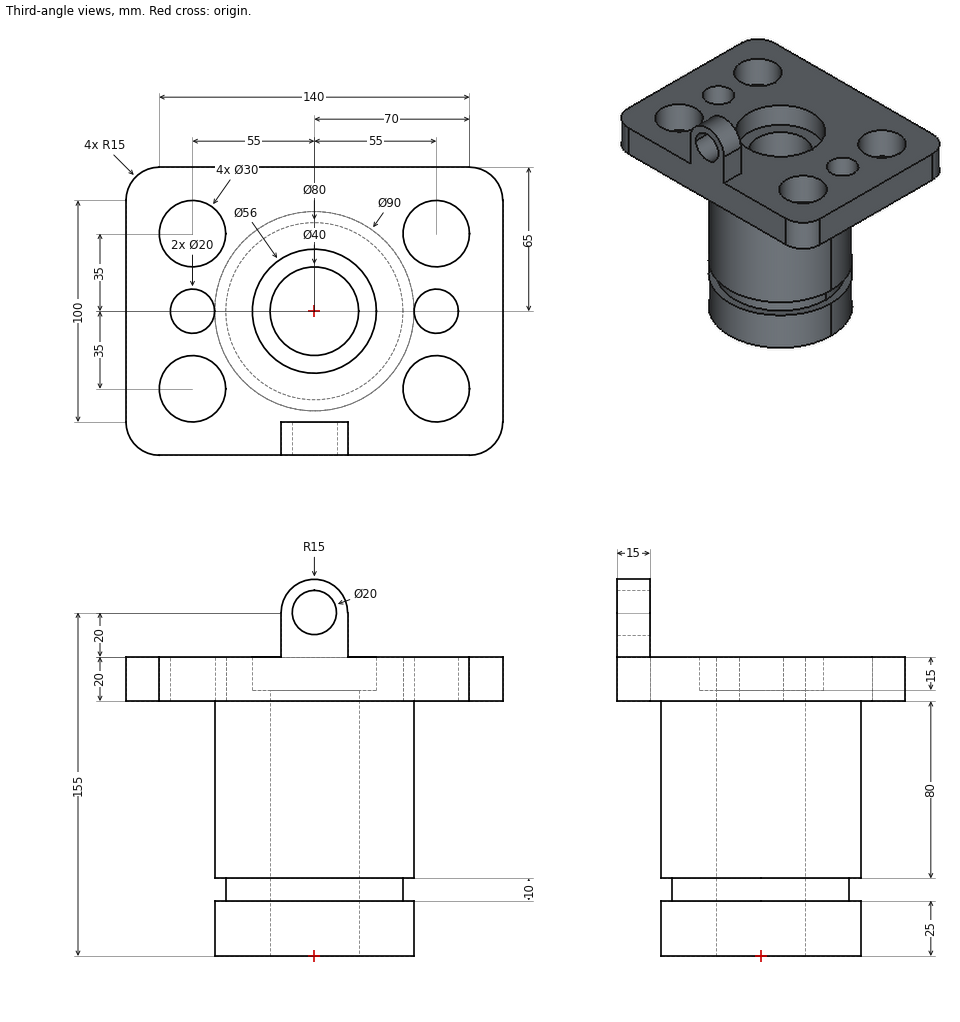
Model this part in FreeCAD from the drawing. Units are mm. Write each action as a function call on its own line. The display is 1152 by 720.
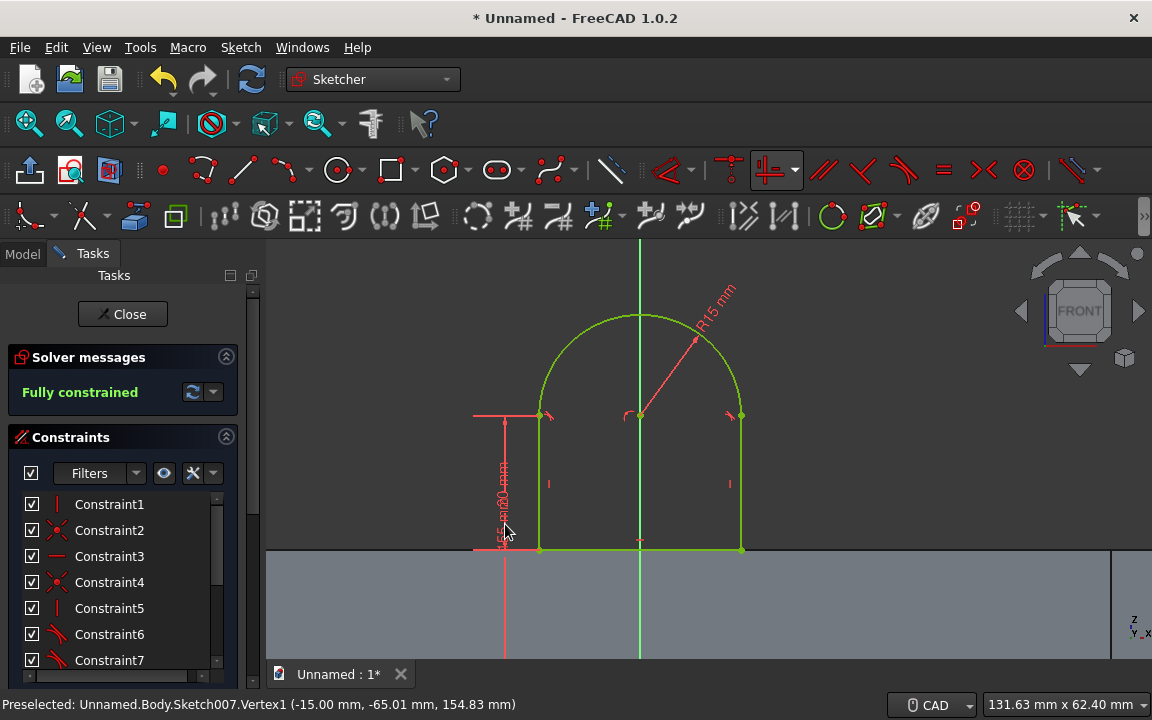
click(123, 314)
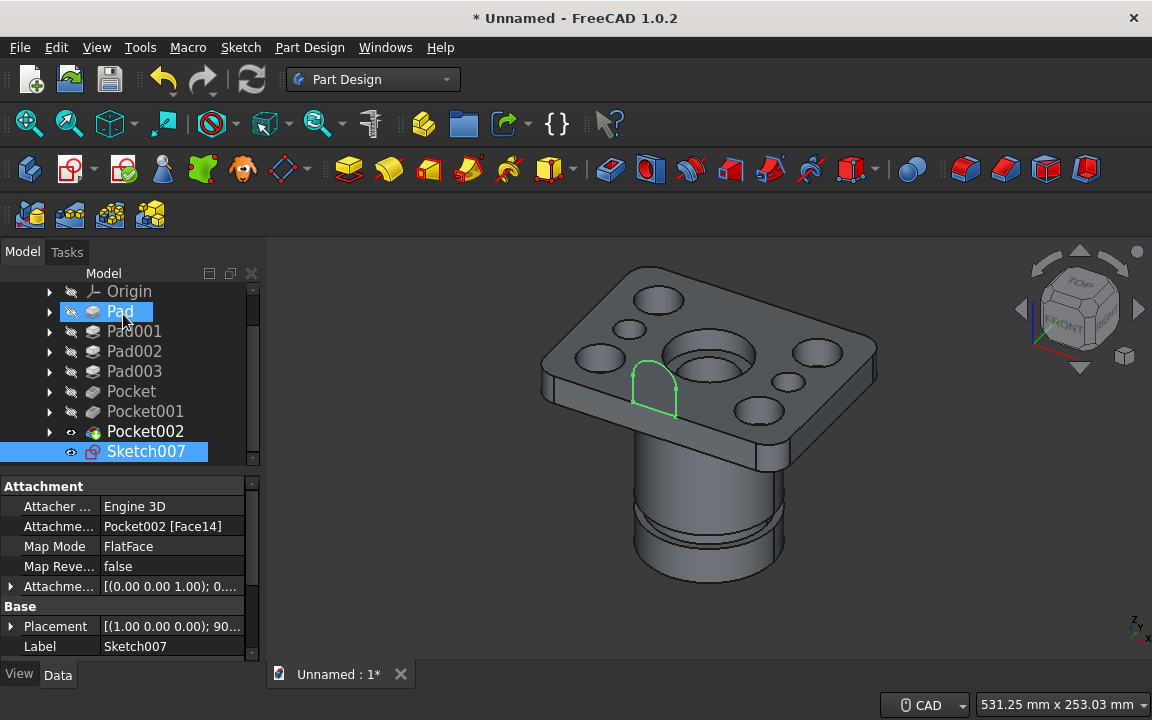
click(350, 170)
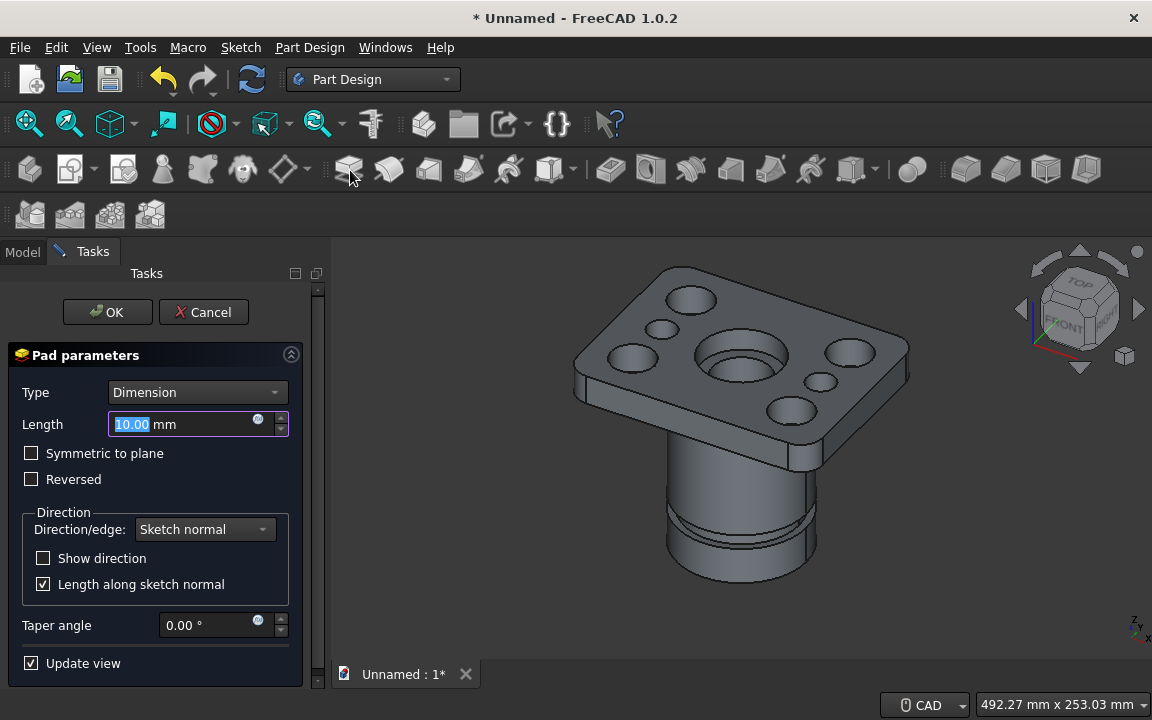
text(15)
key(Tab)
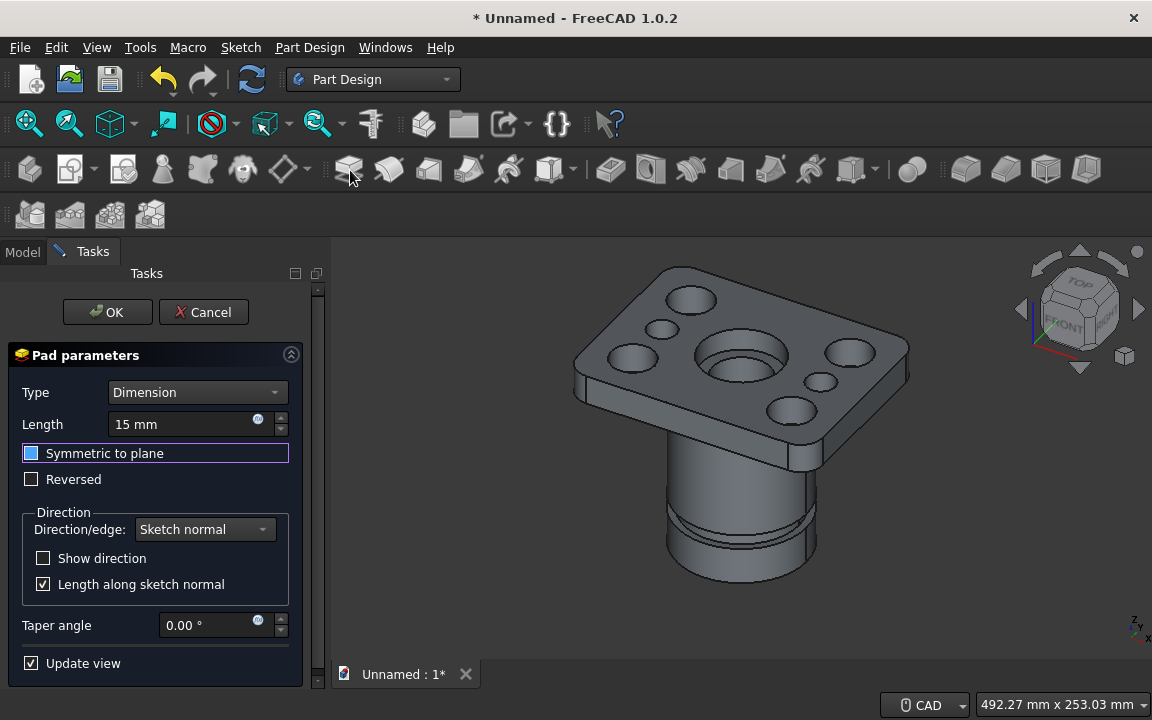
click(30, 479)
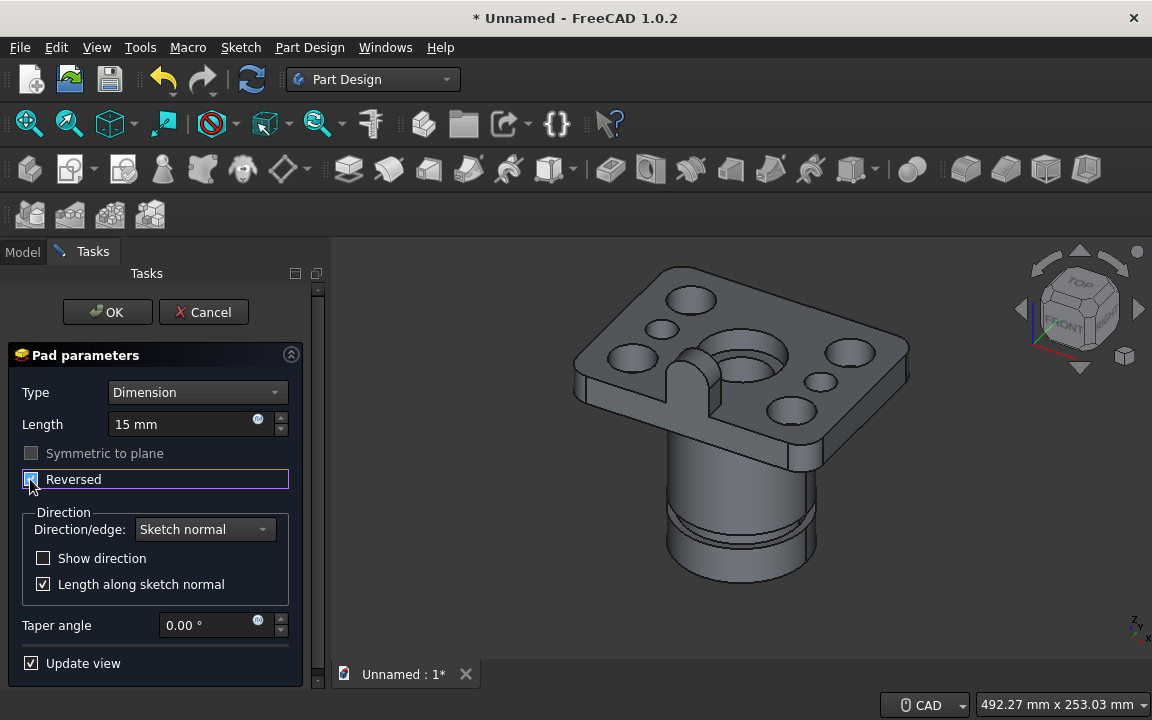
click(108, 312)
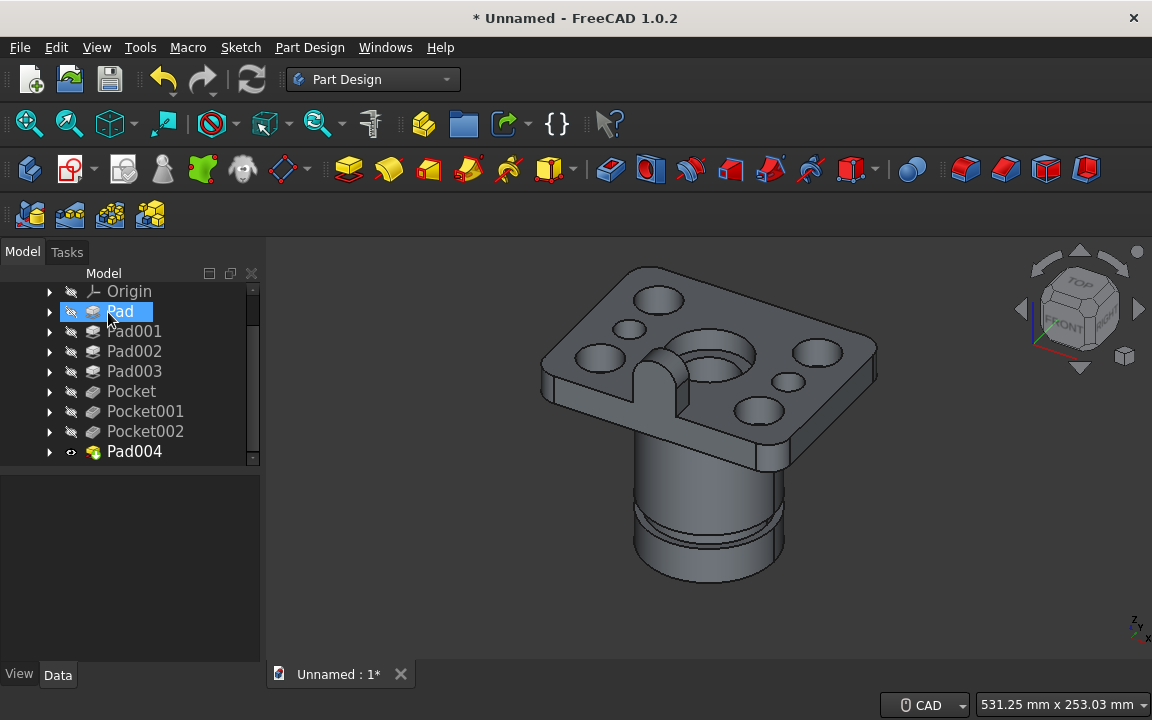
click(30, 124)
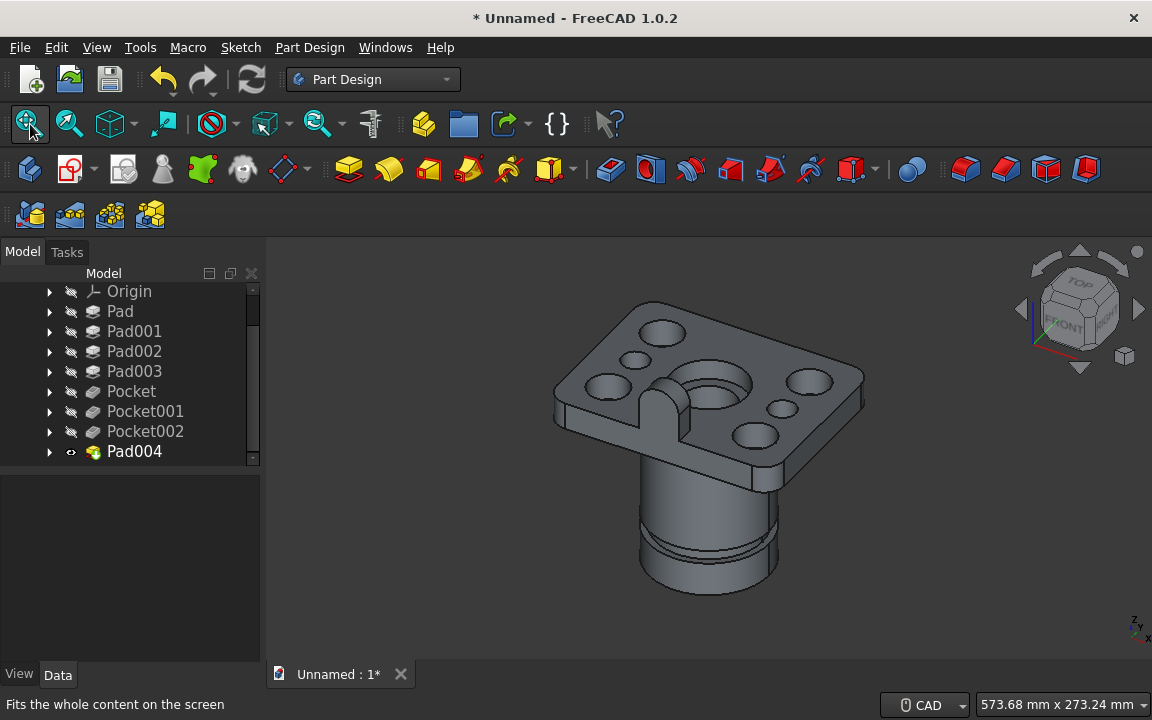
key(4)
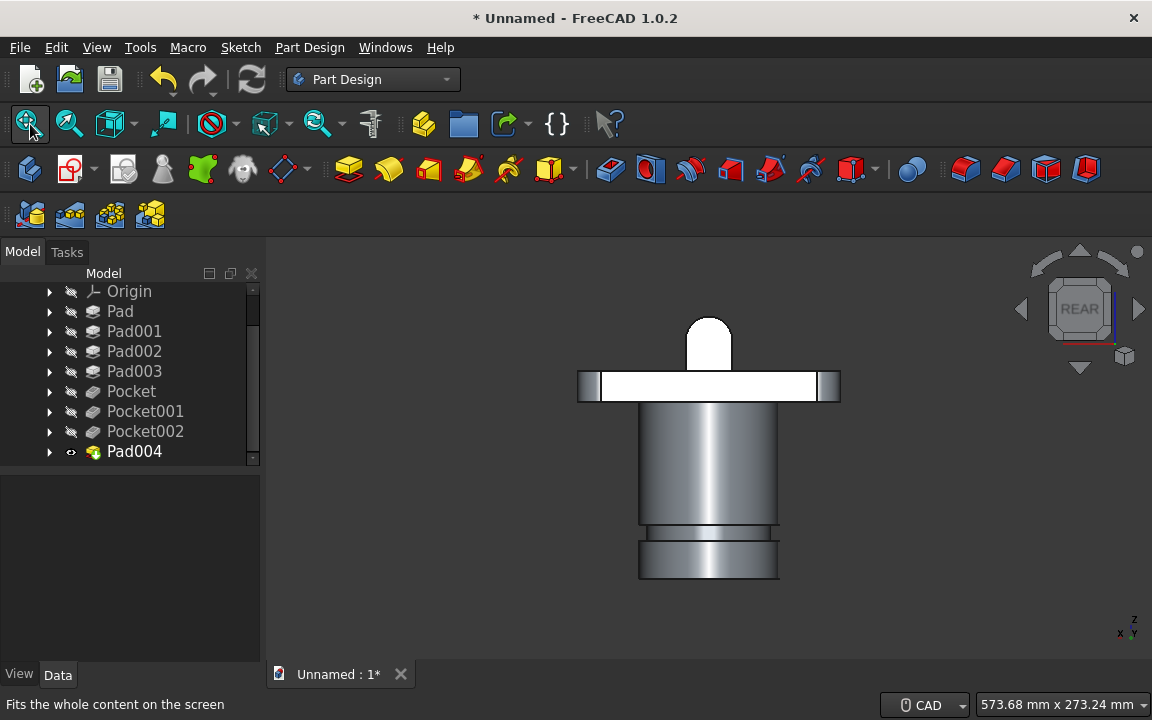
click(709, 343)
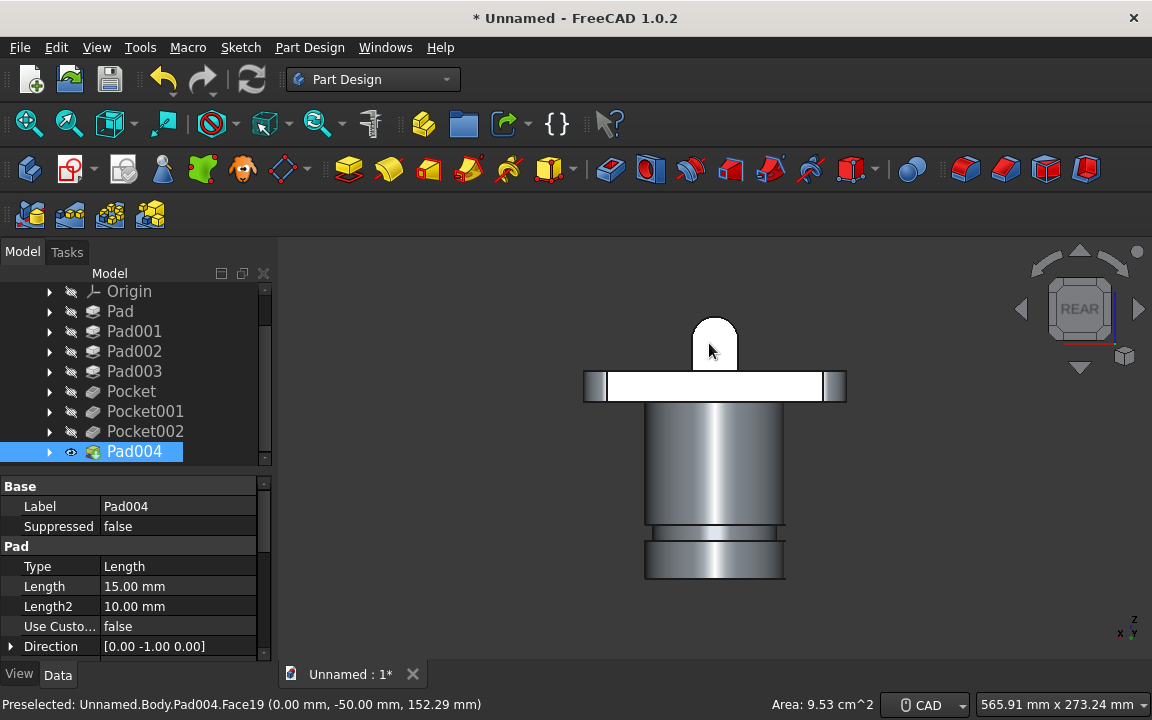
click(70, 170)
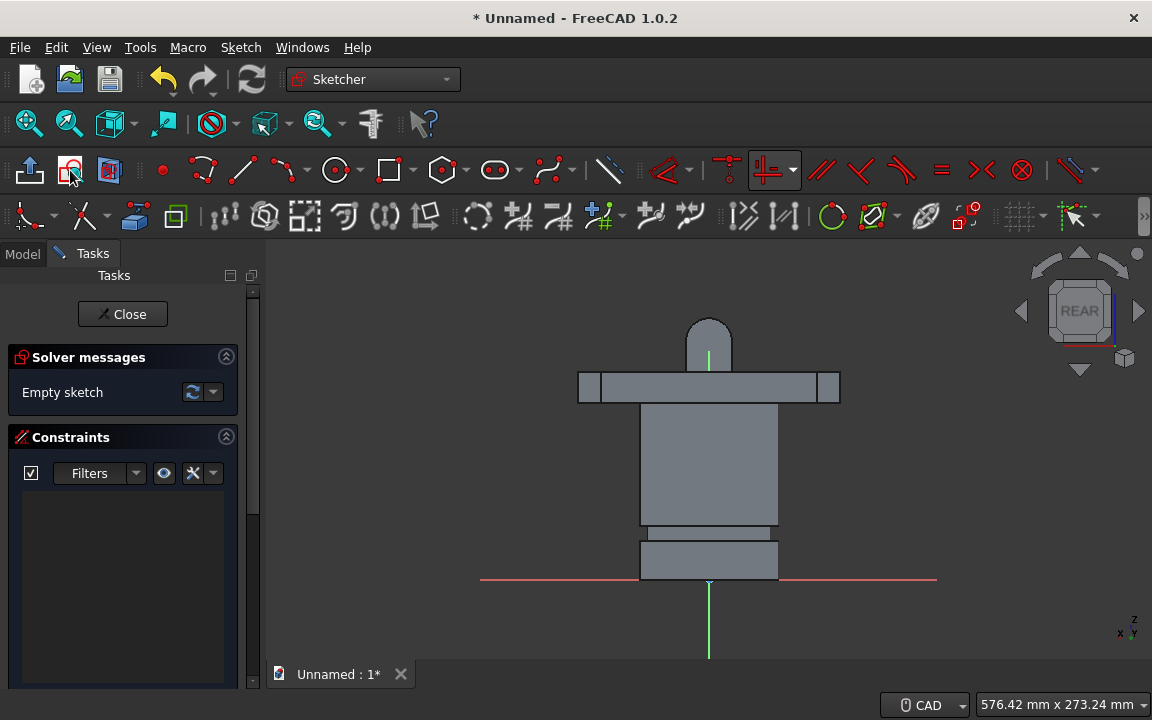
scroll(718, 328, up, 11)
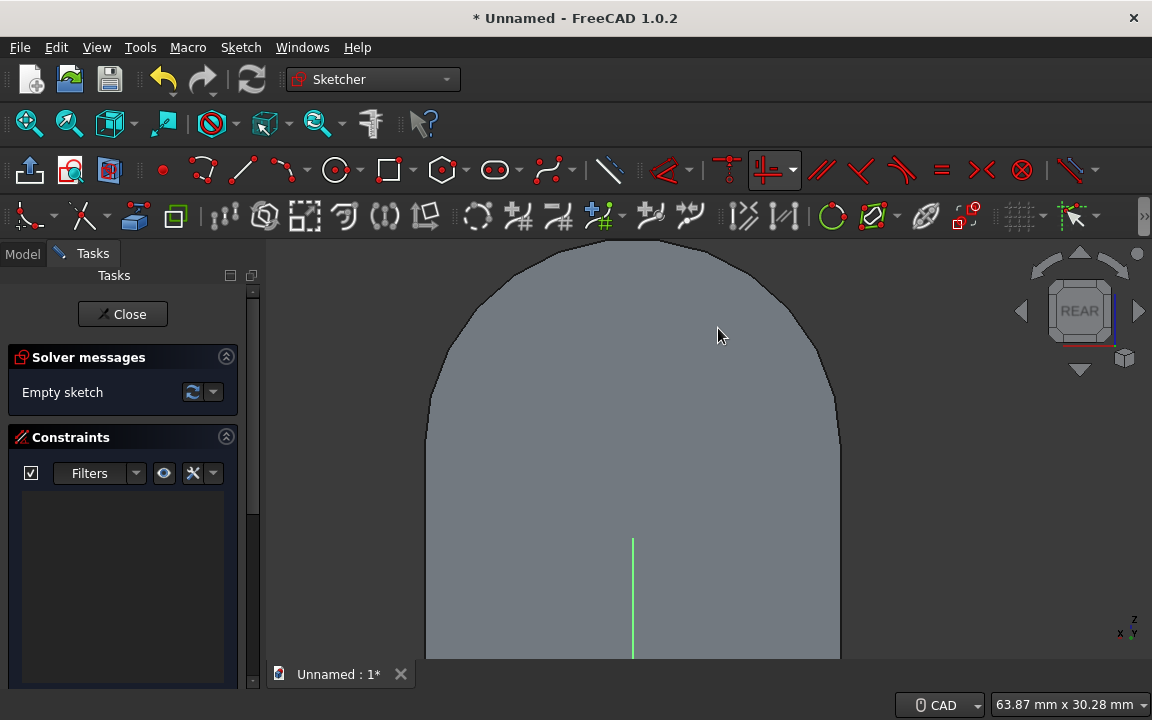
click(336, 170)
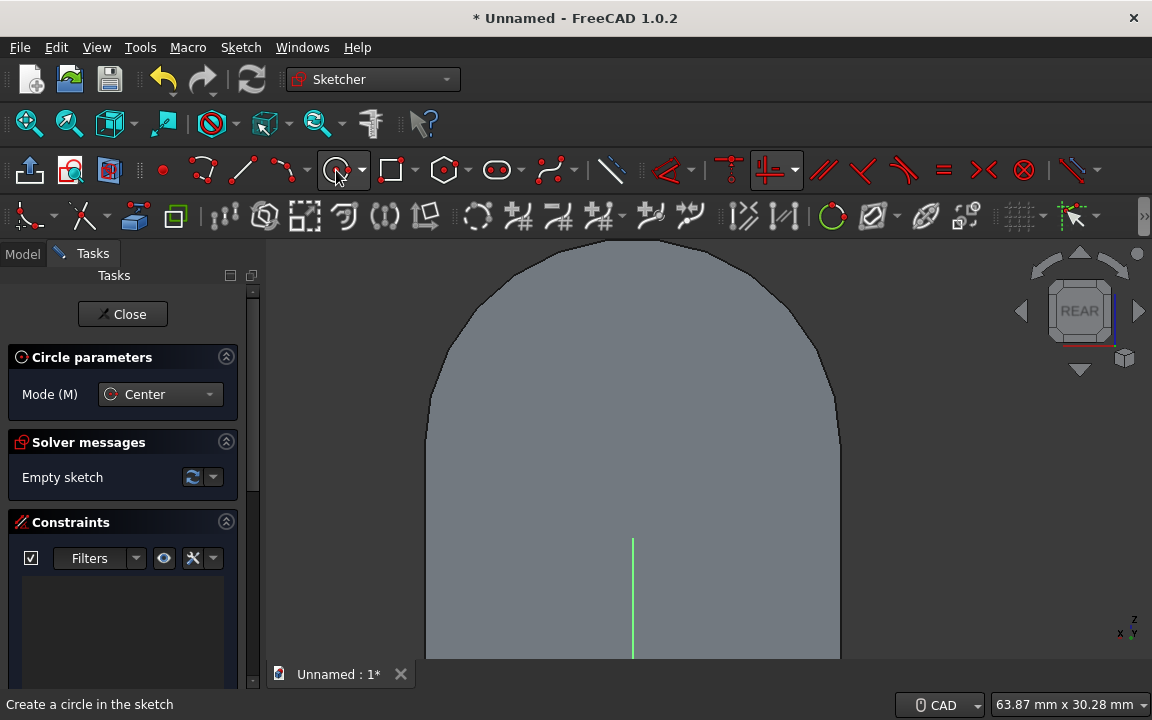
click(633, 447)
click(731, 348)
key(Escape)